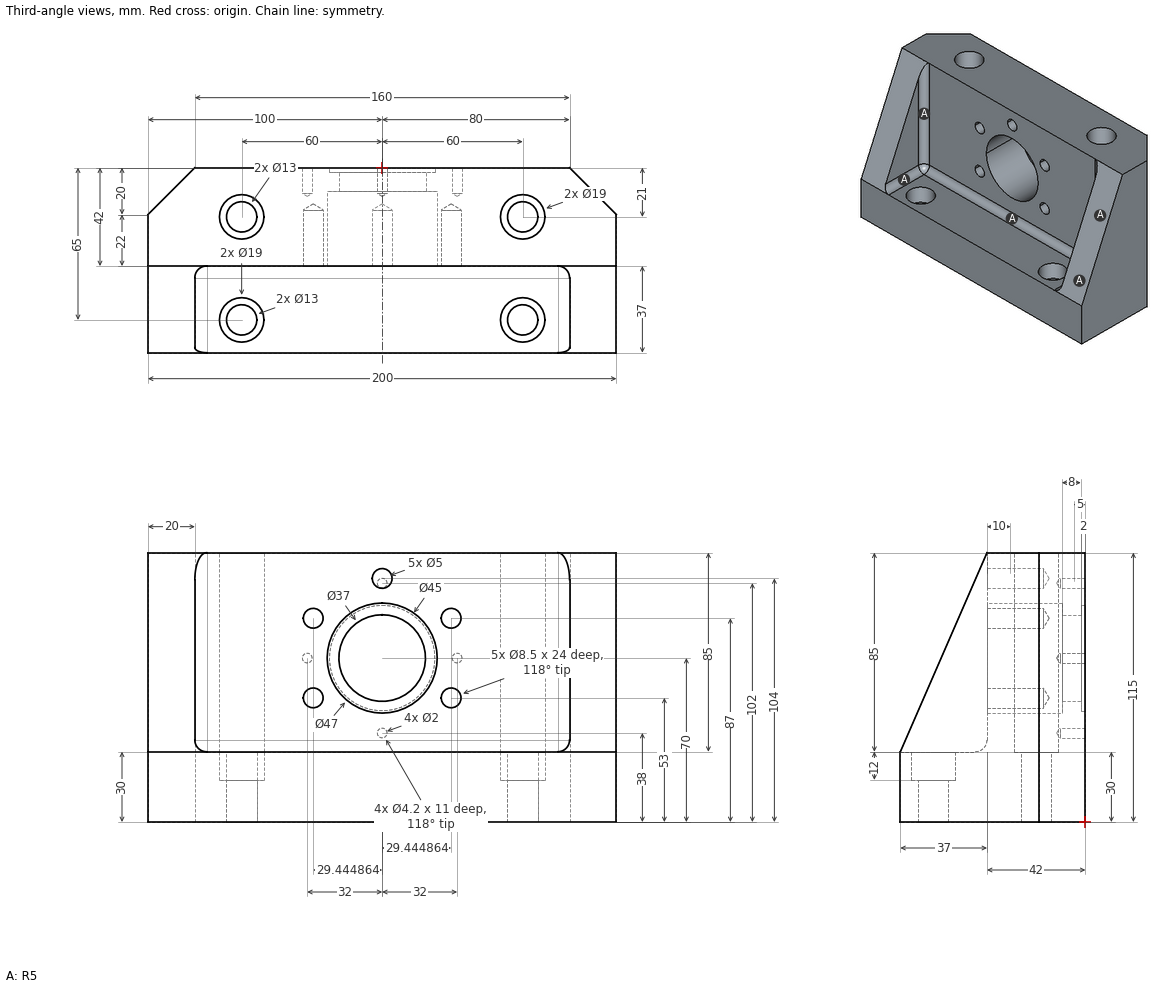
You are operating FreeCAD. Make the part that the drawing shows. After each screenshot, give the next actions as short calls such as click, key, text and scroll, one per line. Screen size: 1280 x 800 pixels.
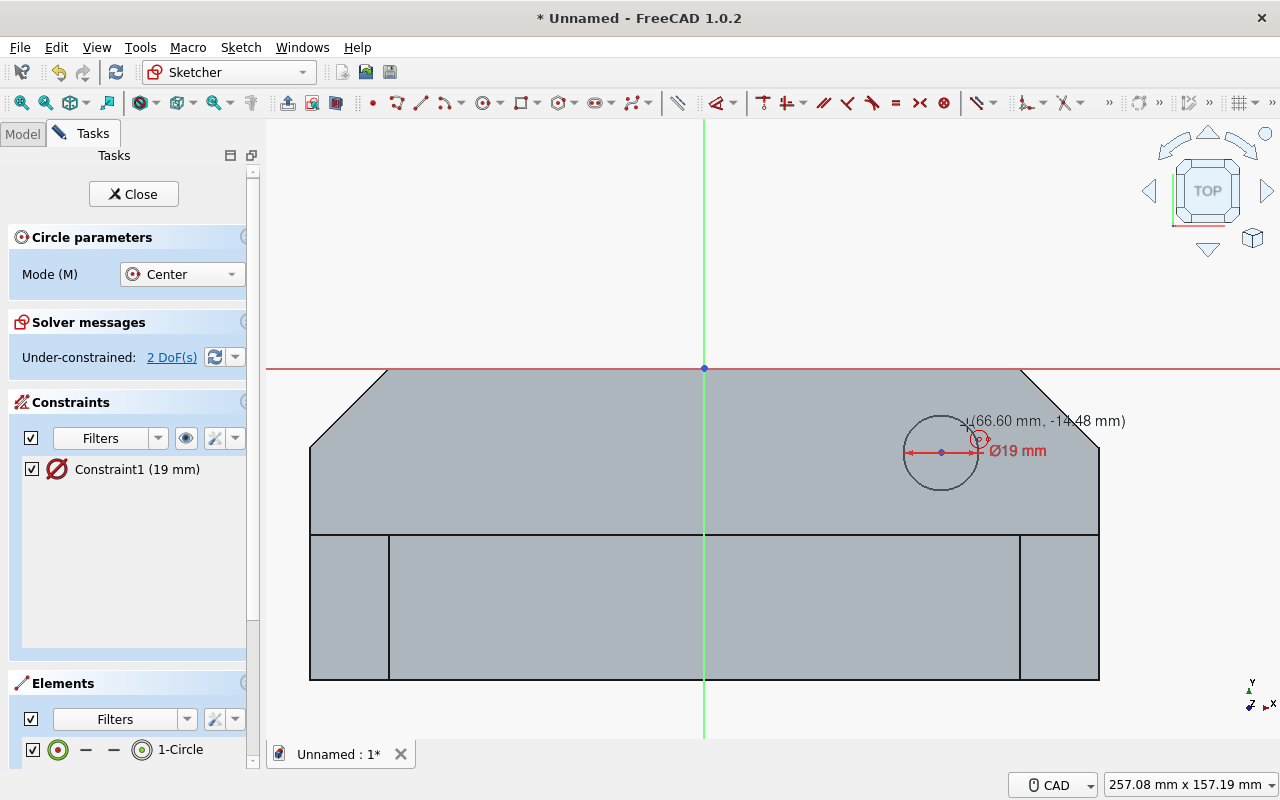
click(468, 452)
move(494, 425)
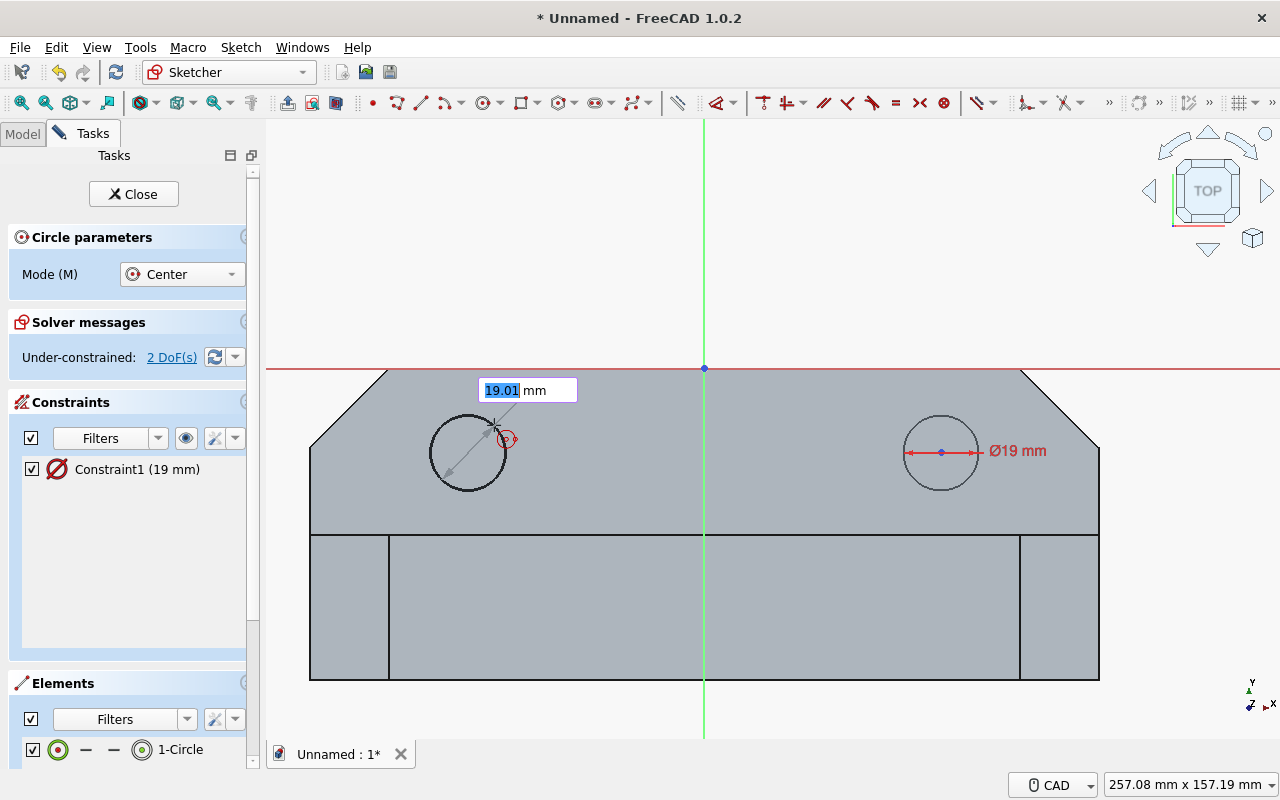
text(19)
key(Return)
key(Escape)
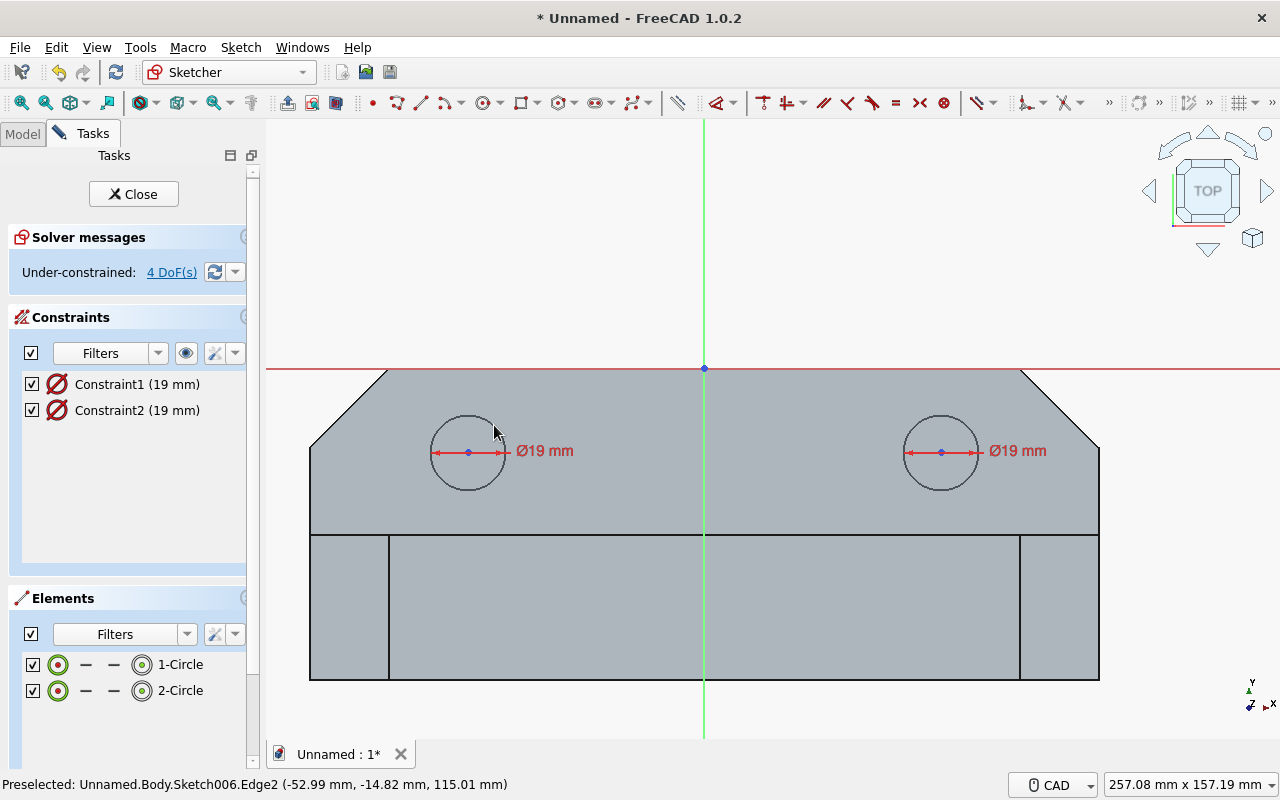
click(941, 453)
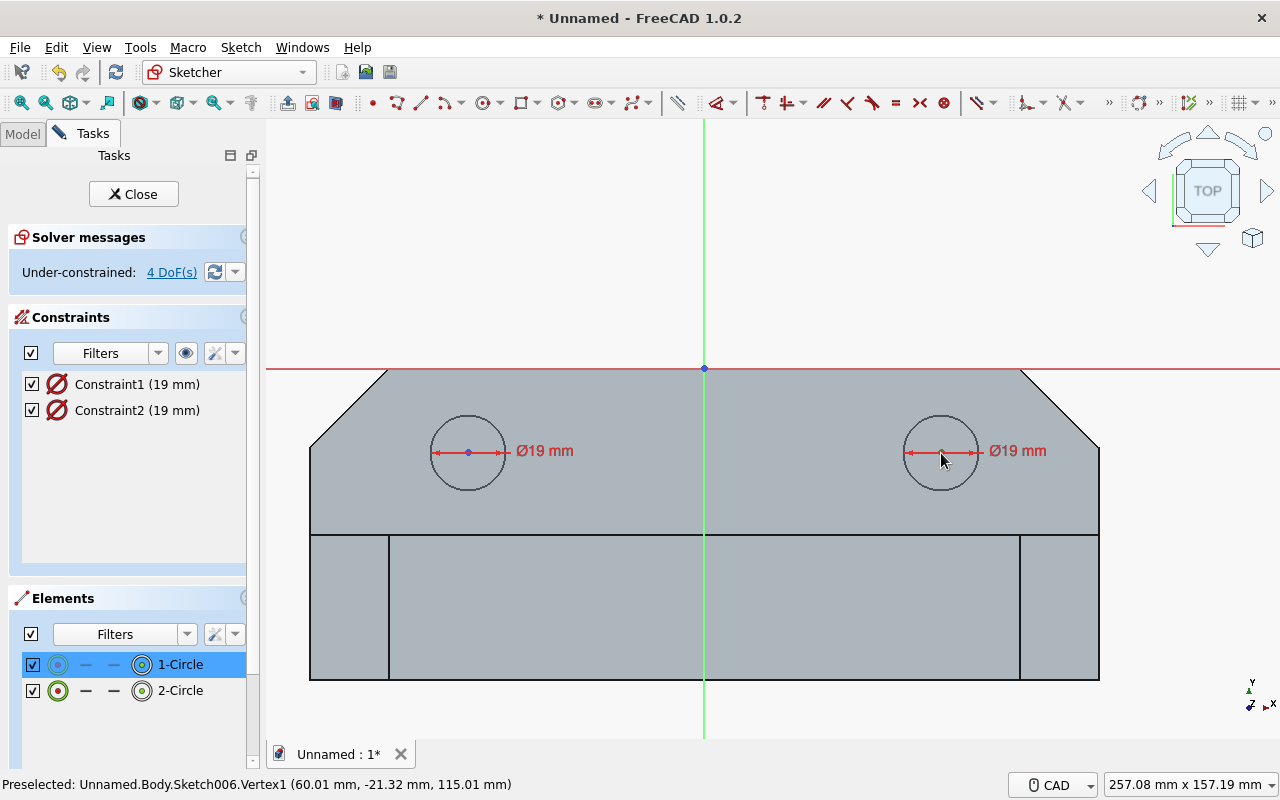
click(468, 453)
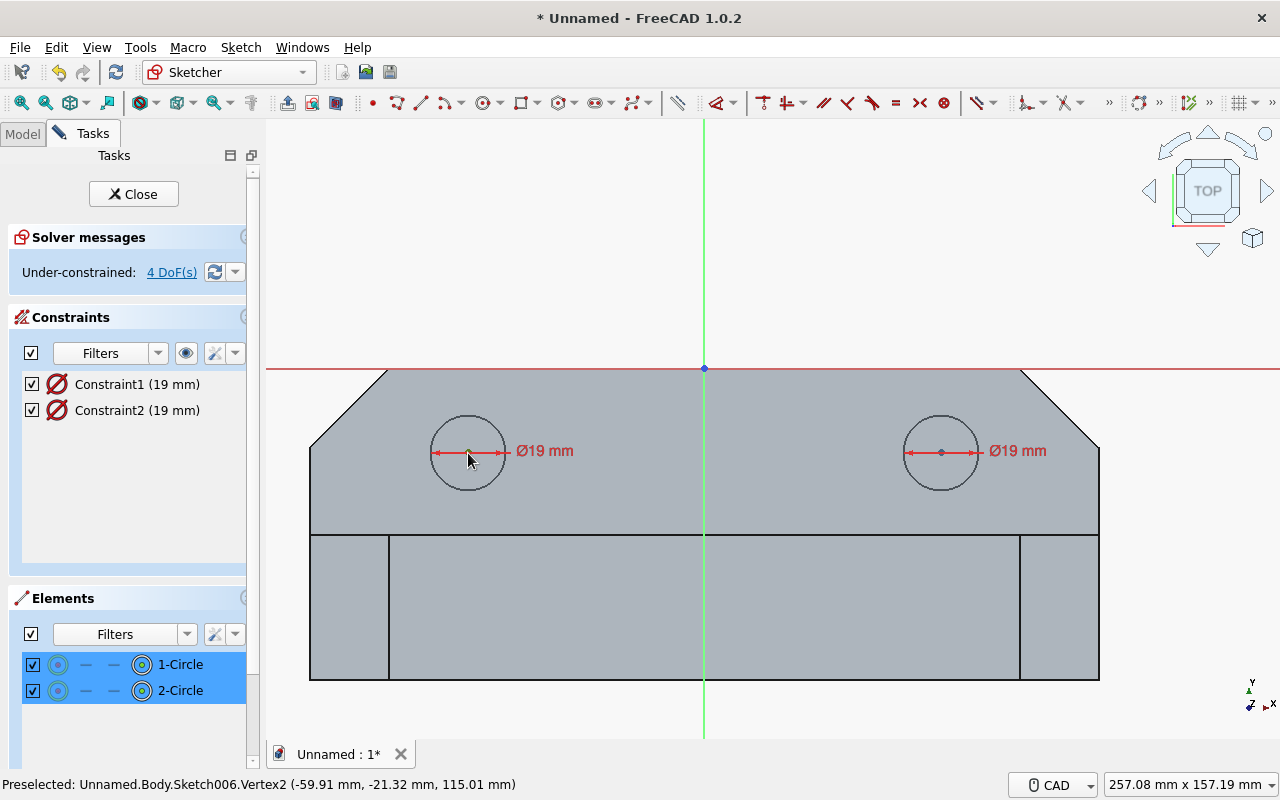
click(806, 104)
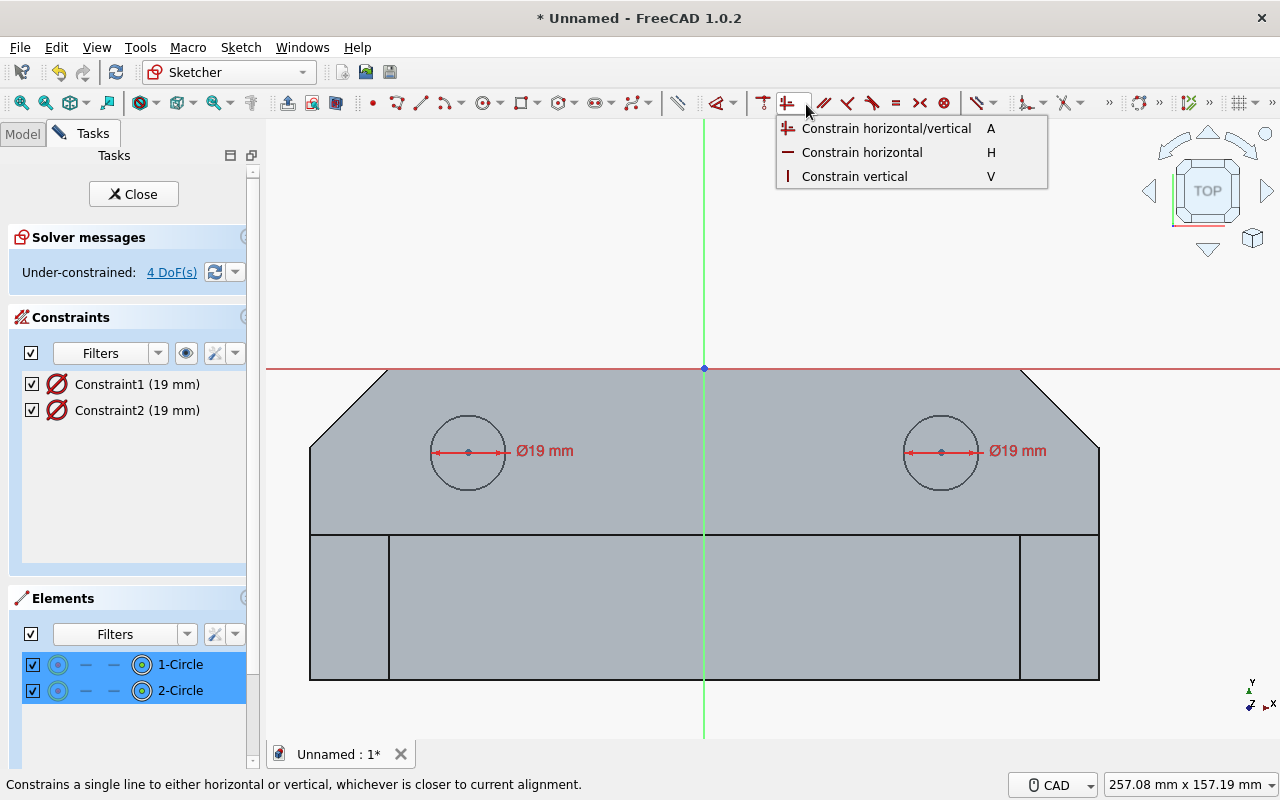
click(912, 152)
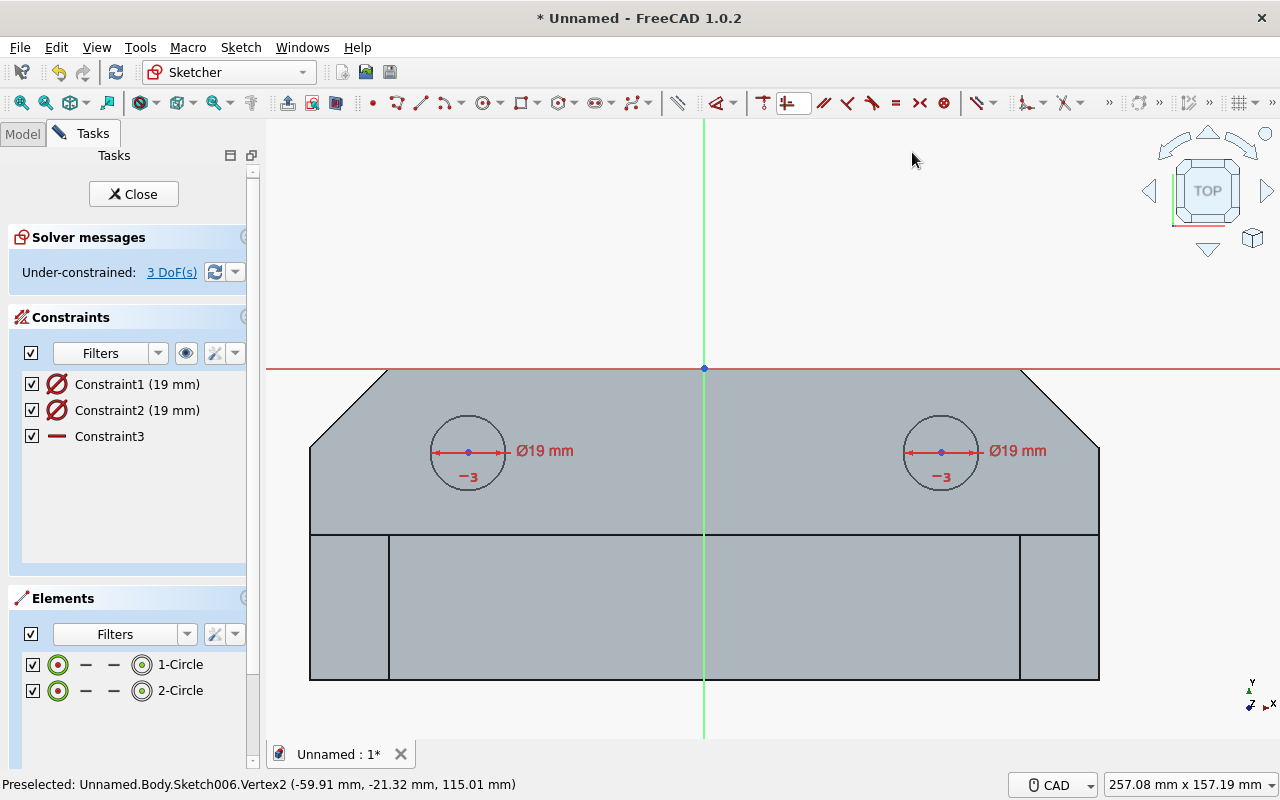
click(716, 104)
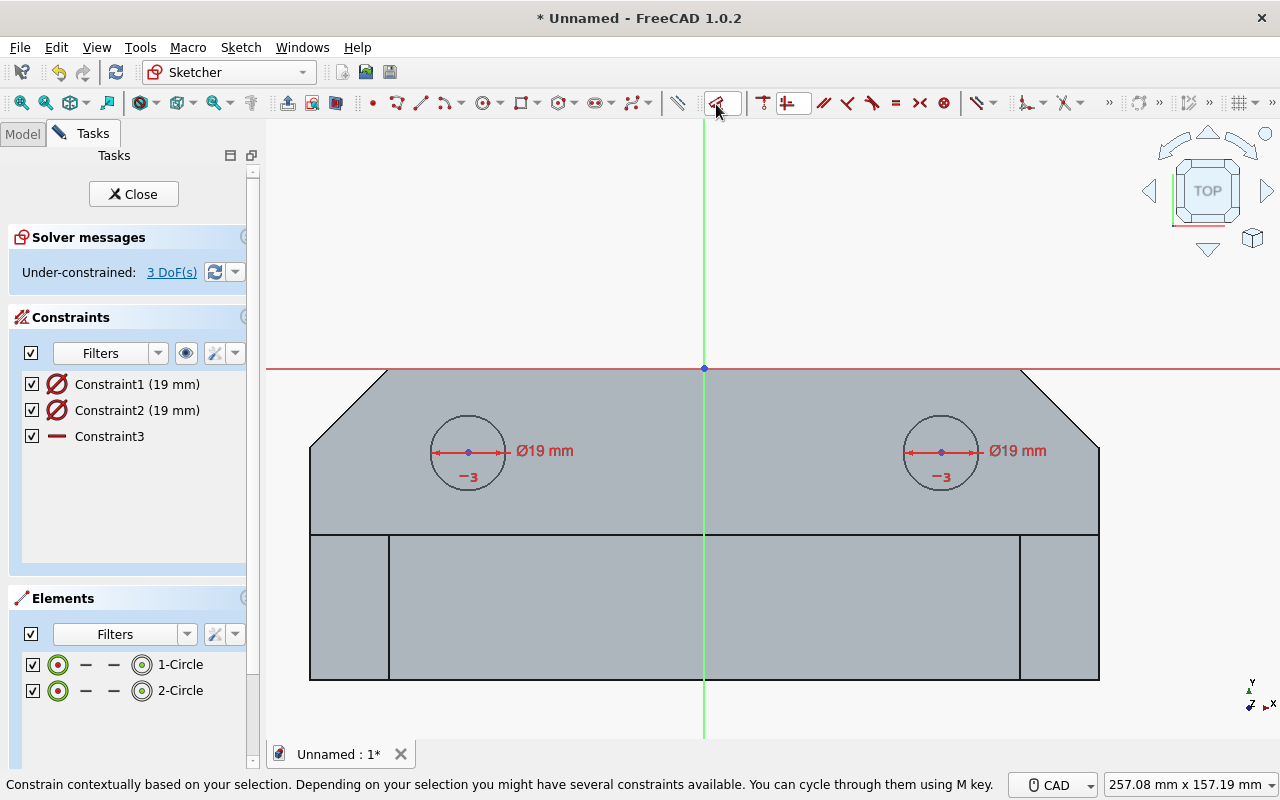
click(941, 453)
click(823, 335)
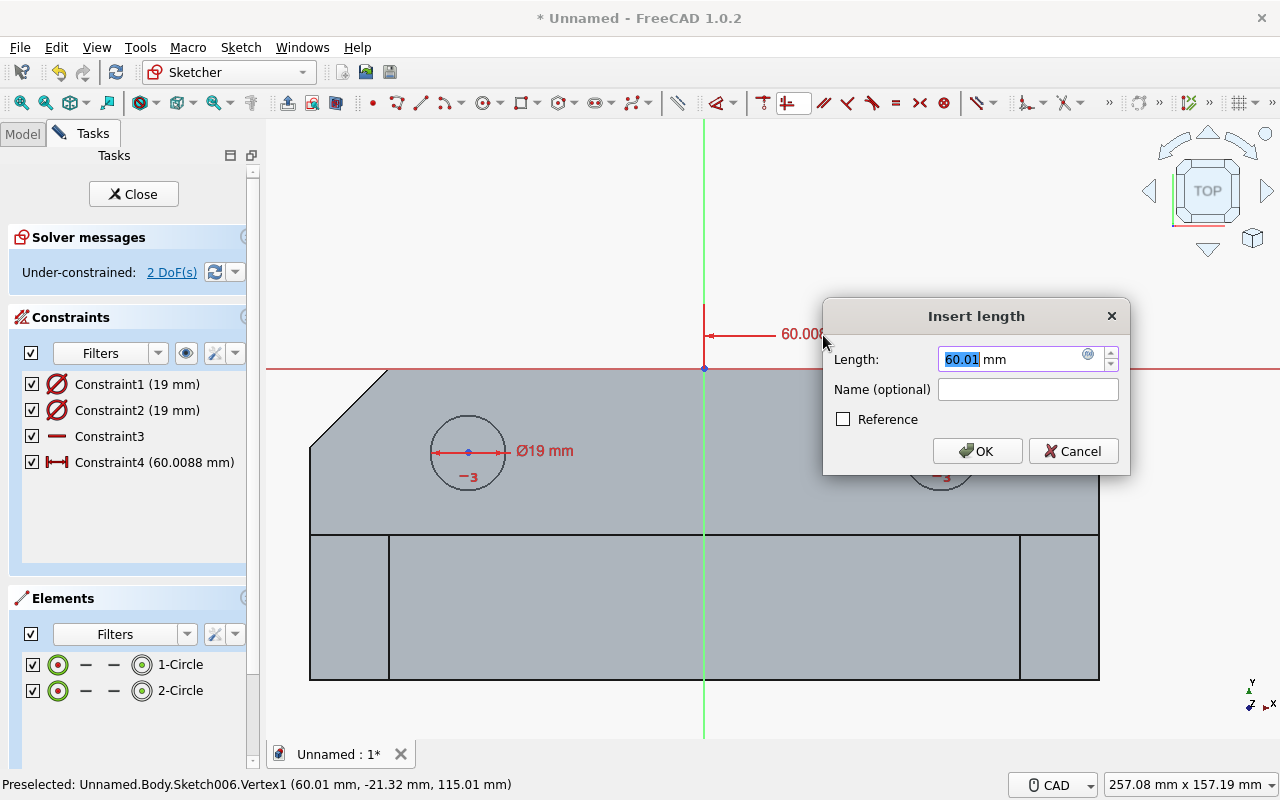
text(60)
key(Return)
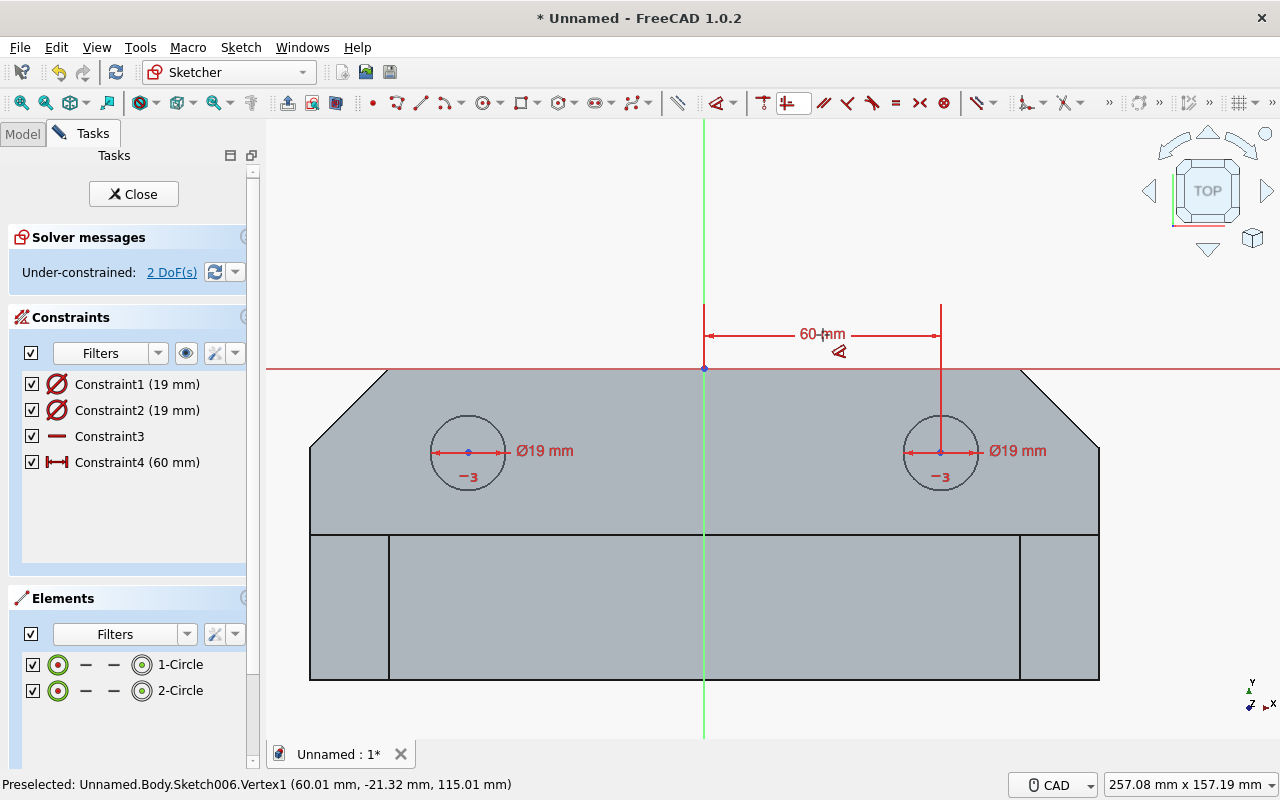
click(941, 453)
click(975, 411)